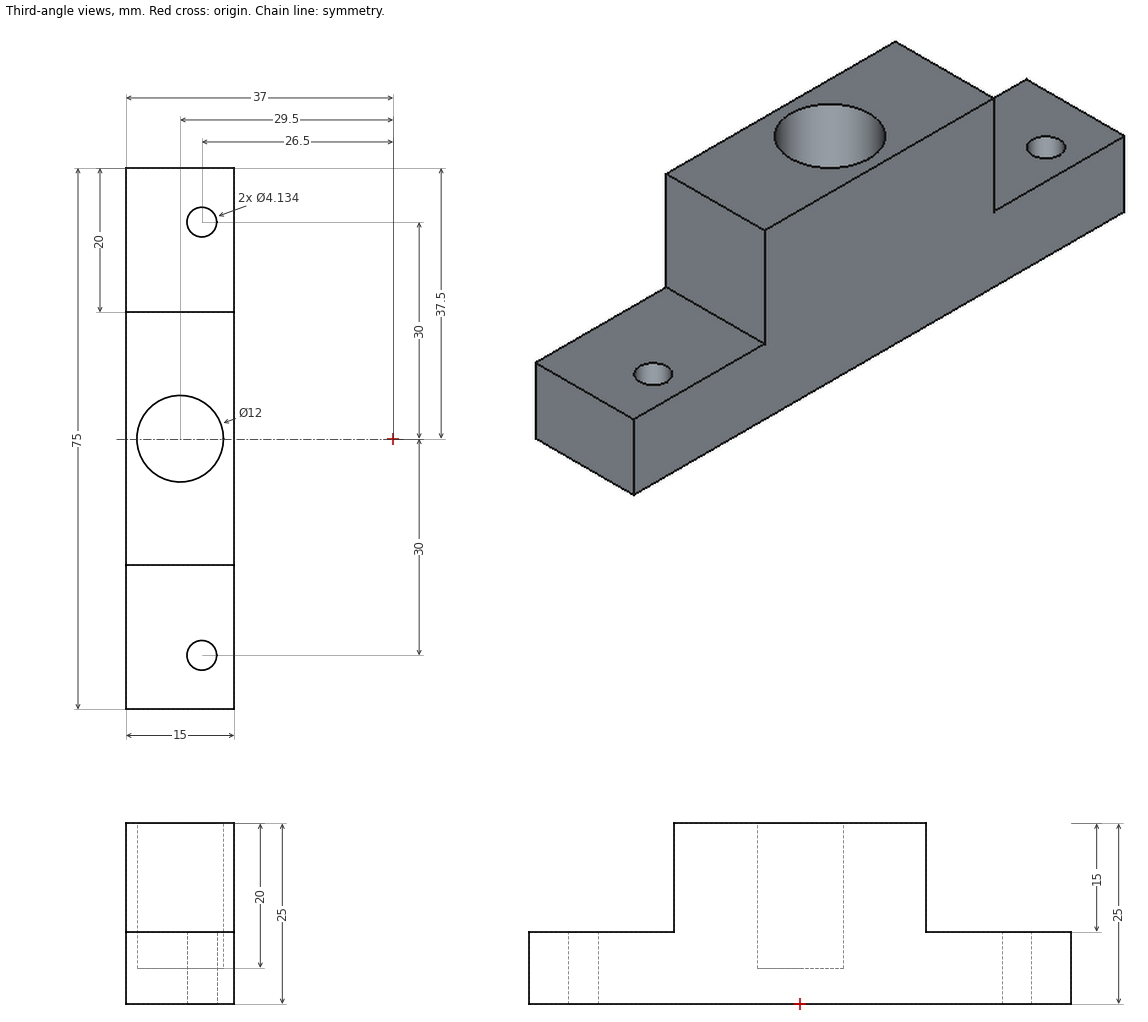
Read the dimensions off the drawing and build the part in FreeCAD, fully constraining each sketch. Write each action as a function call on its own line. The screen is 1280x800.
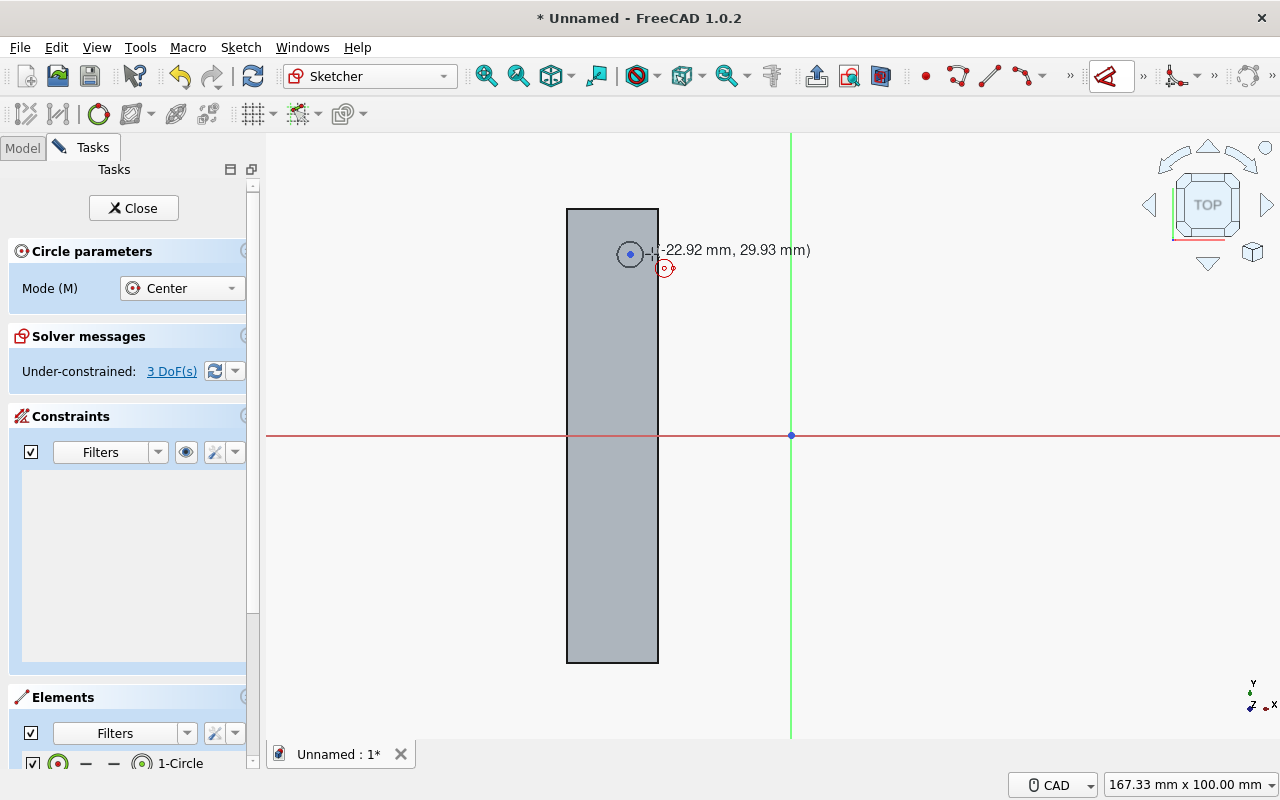
scroll(630, 618, up, 3)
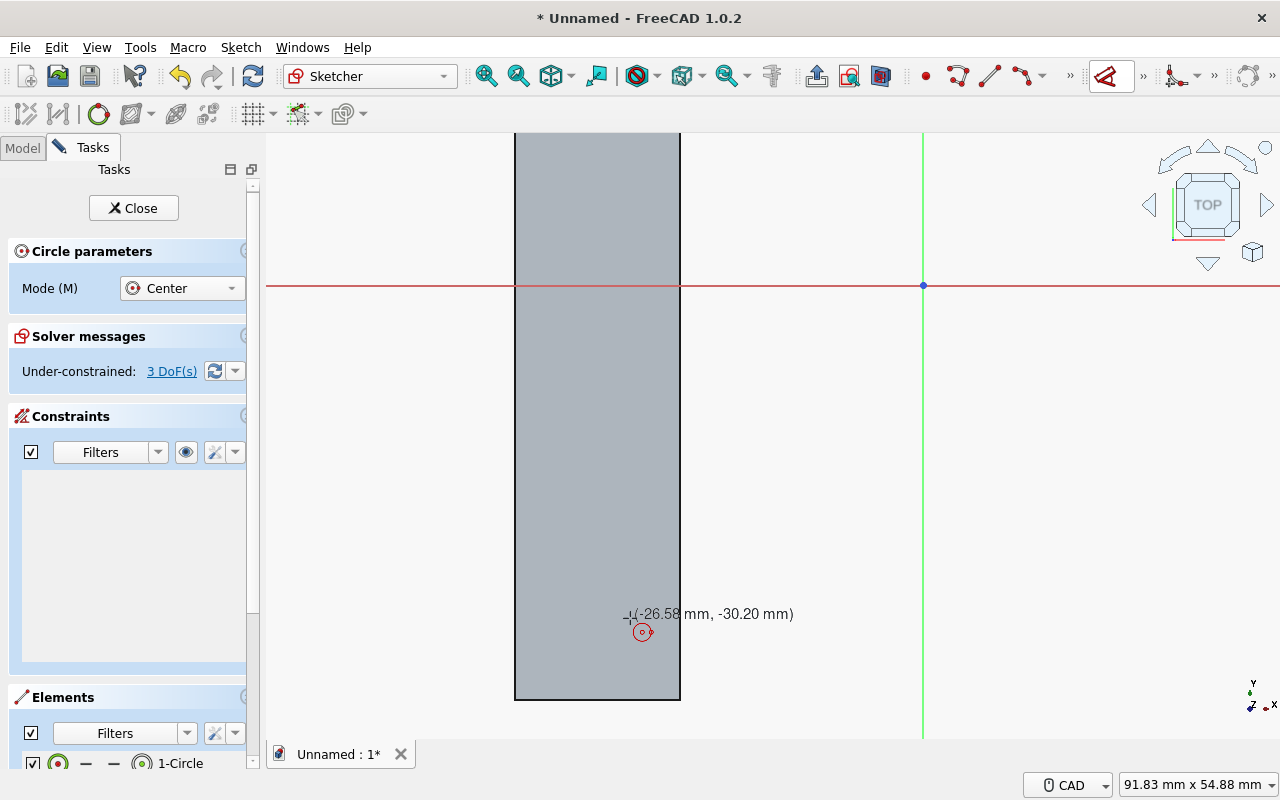
click(631, 617)
click(647, 601)
key(Escape)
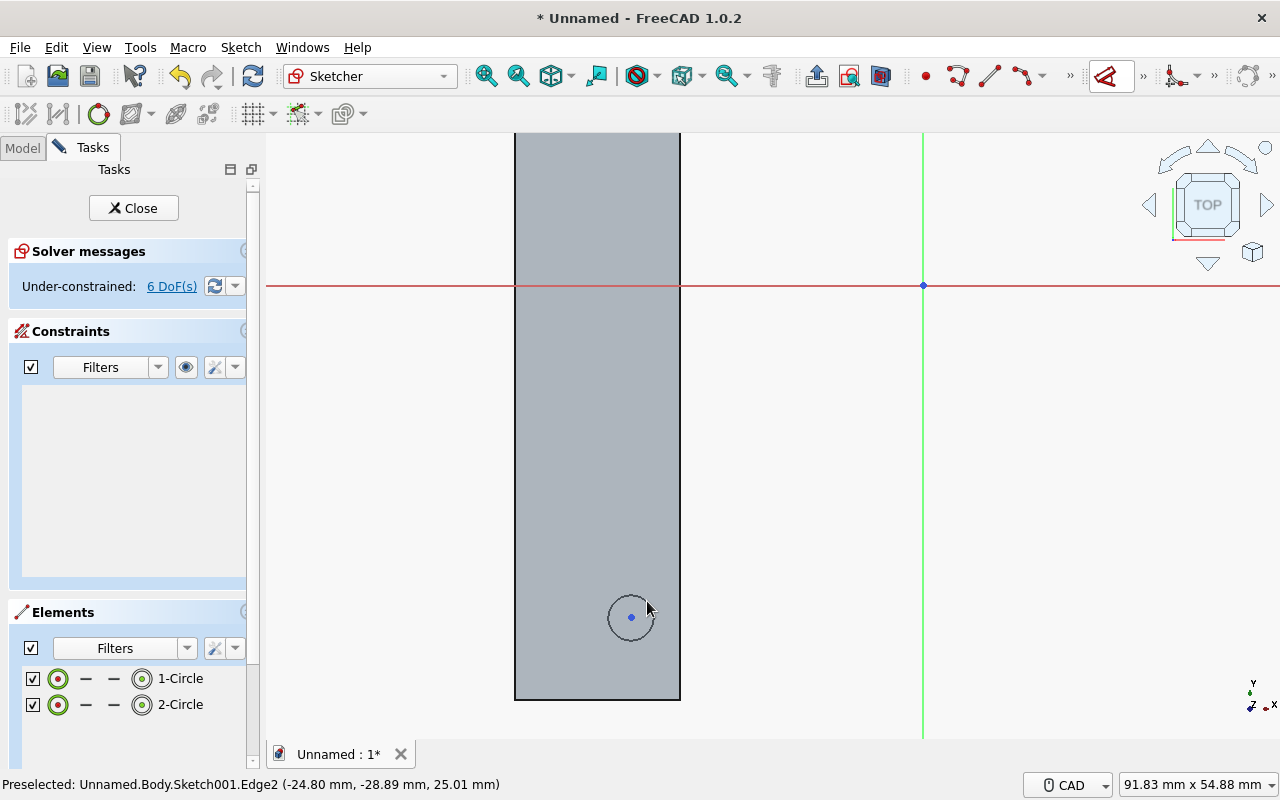
scroll(630, 619, down, 3)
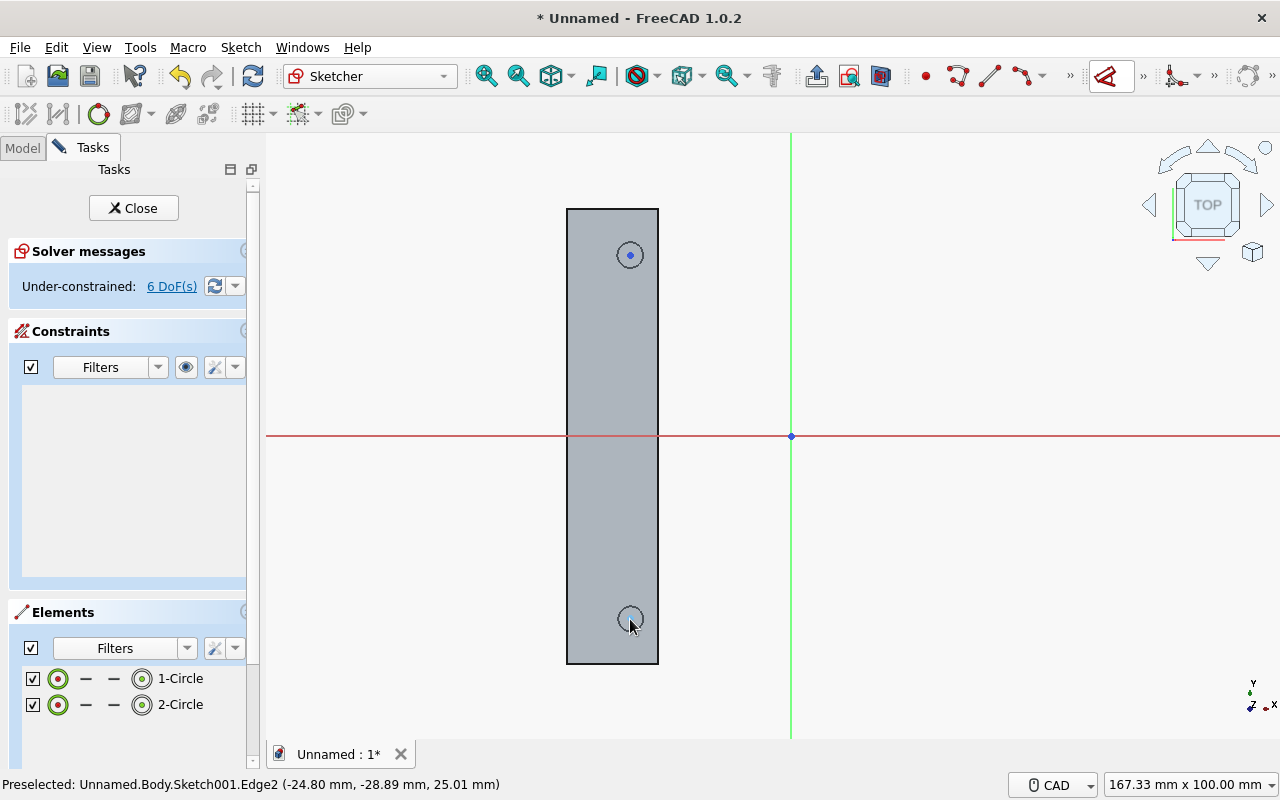
click(639, 246)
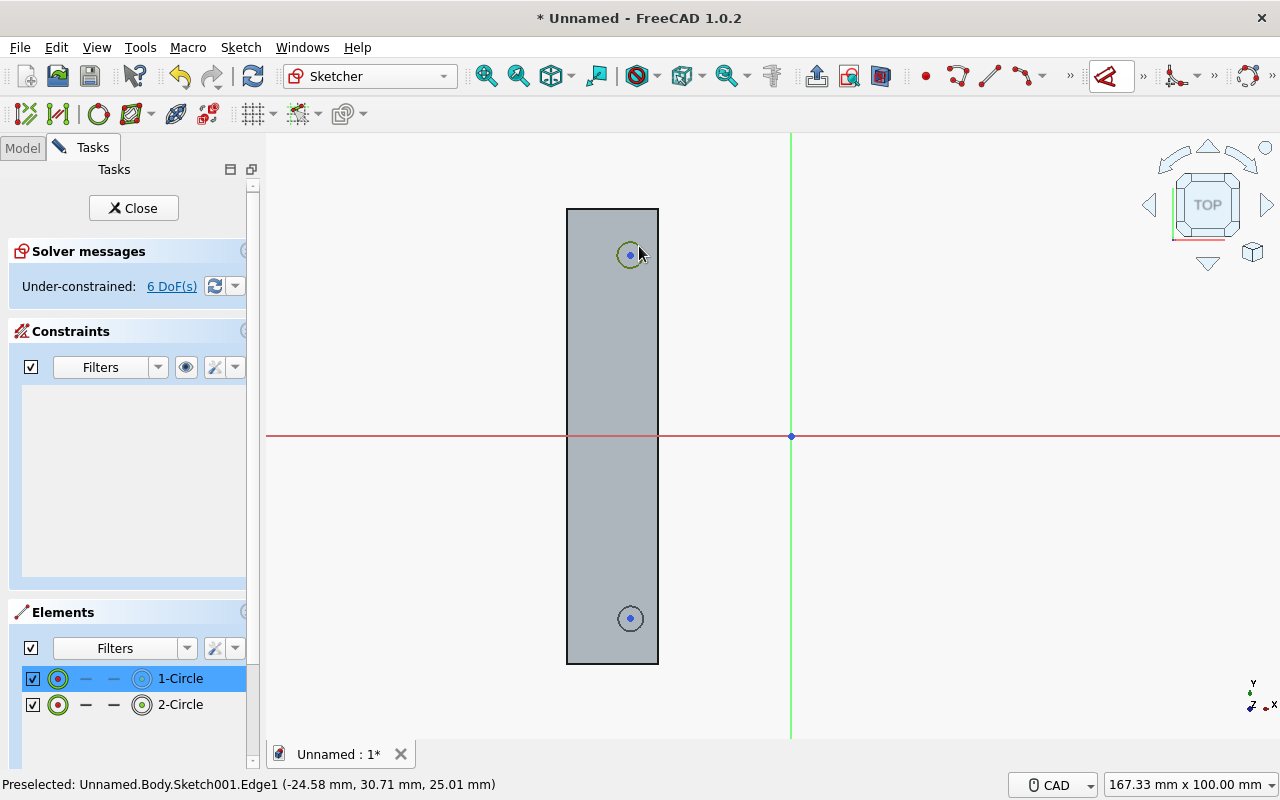
click(639, 610)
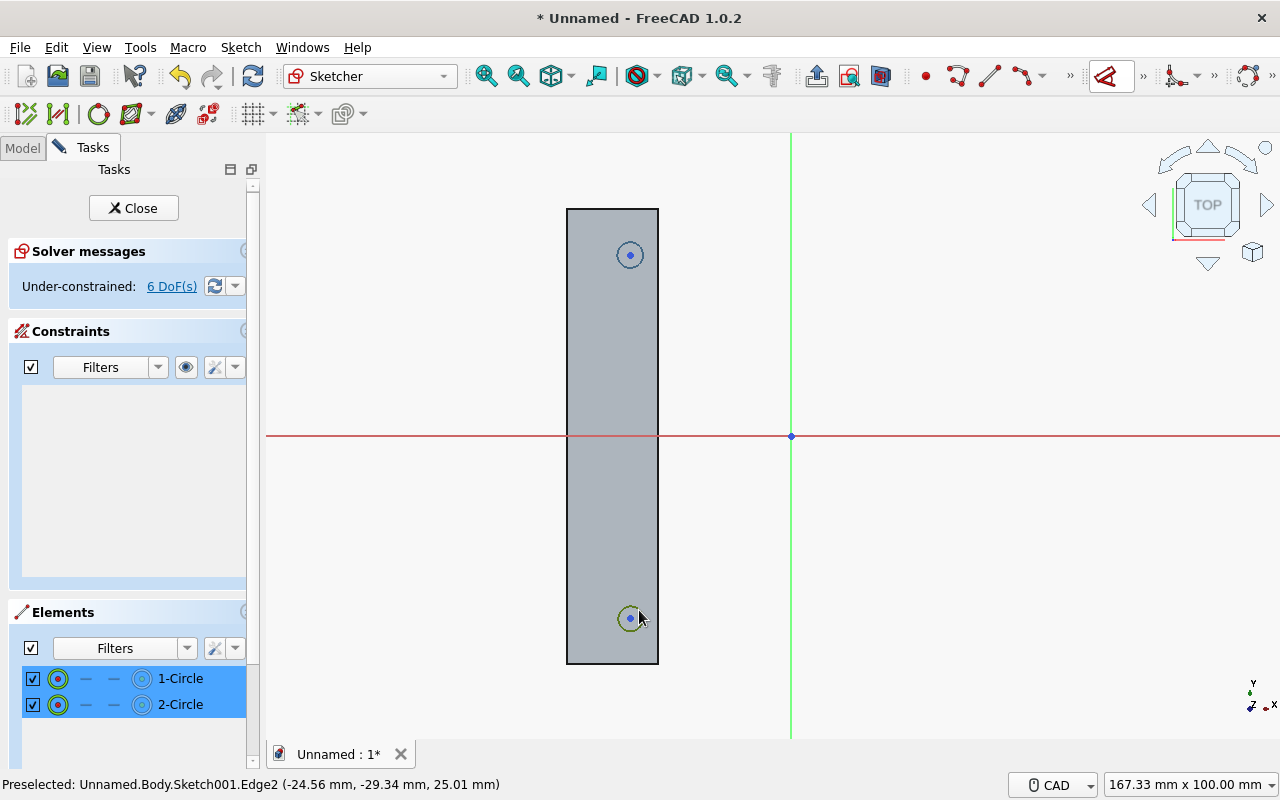
key(e)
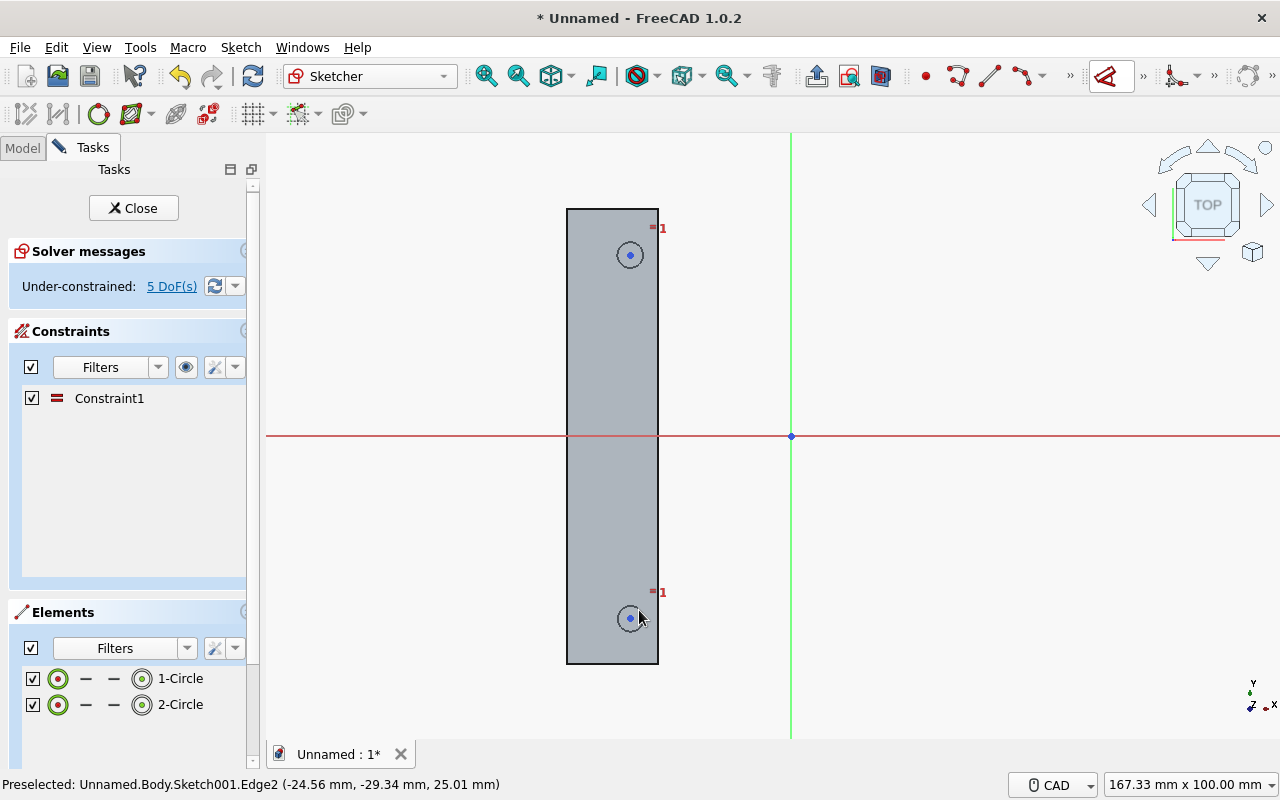
click(630, 255)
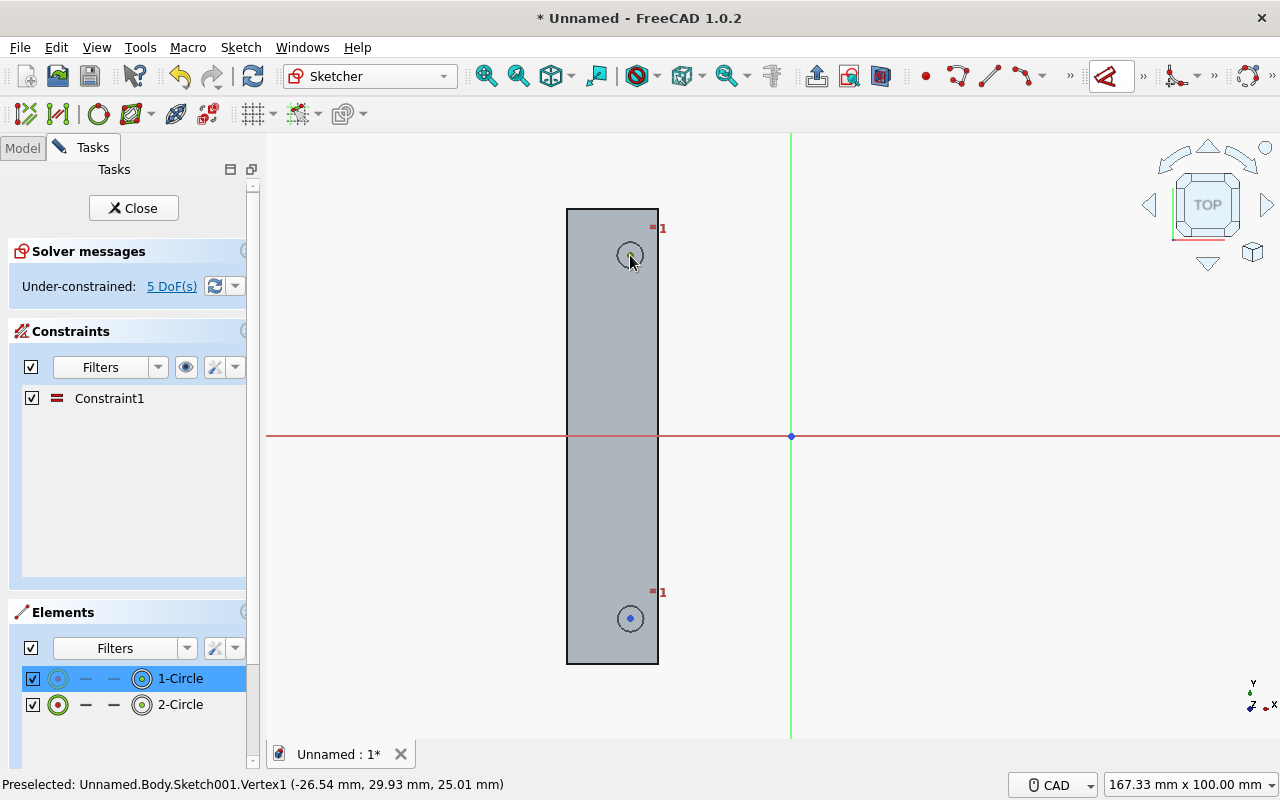
click(631, 619)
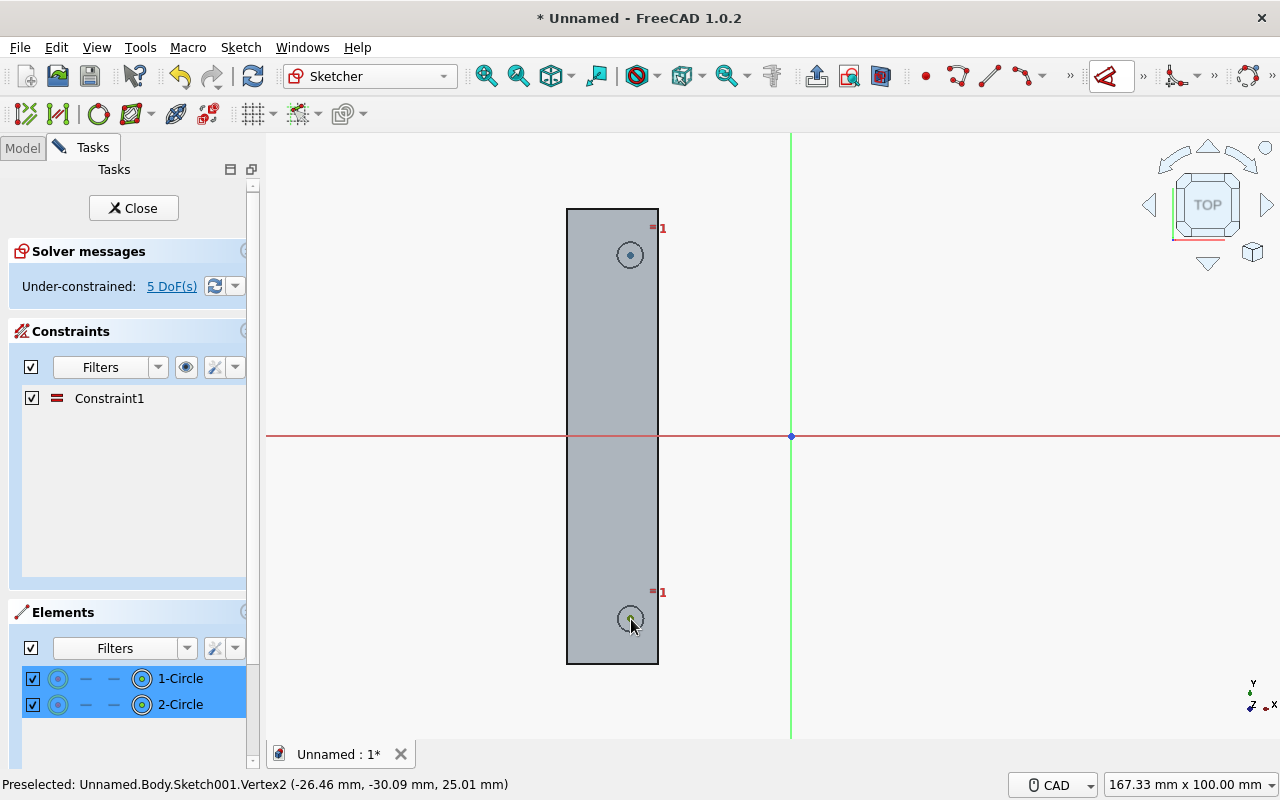
key(v)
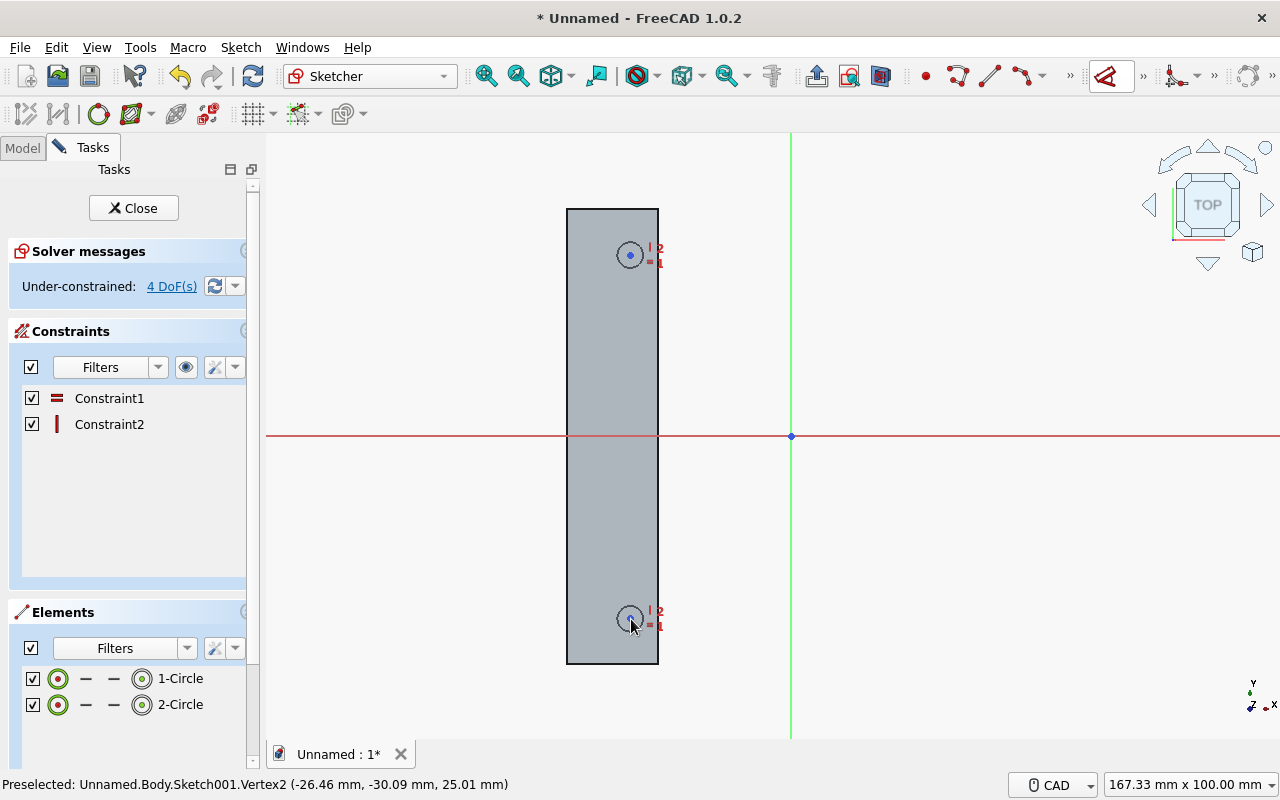
scroll(639, 246, up, 3)